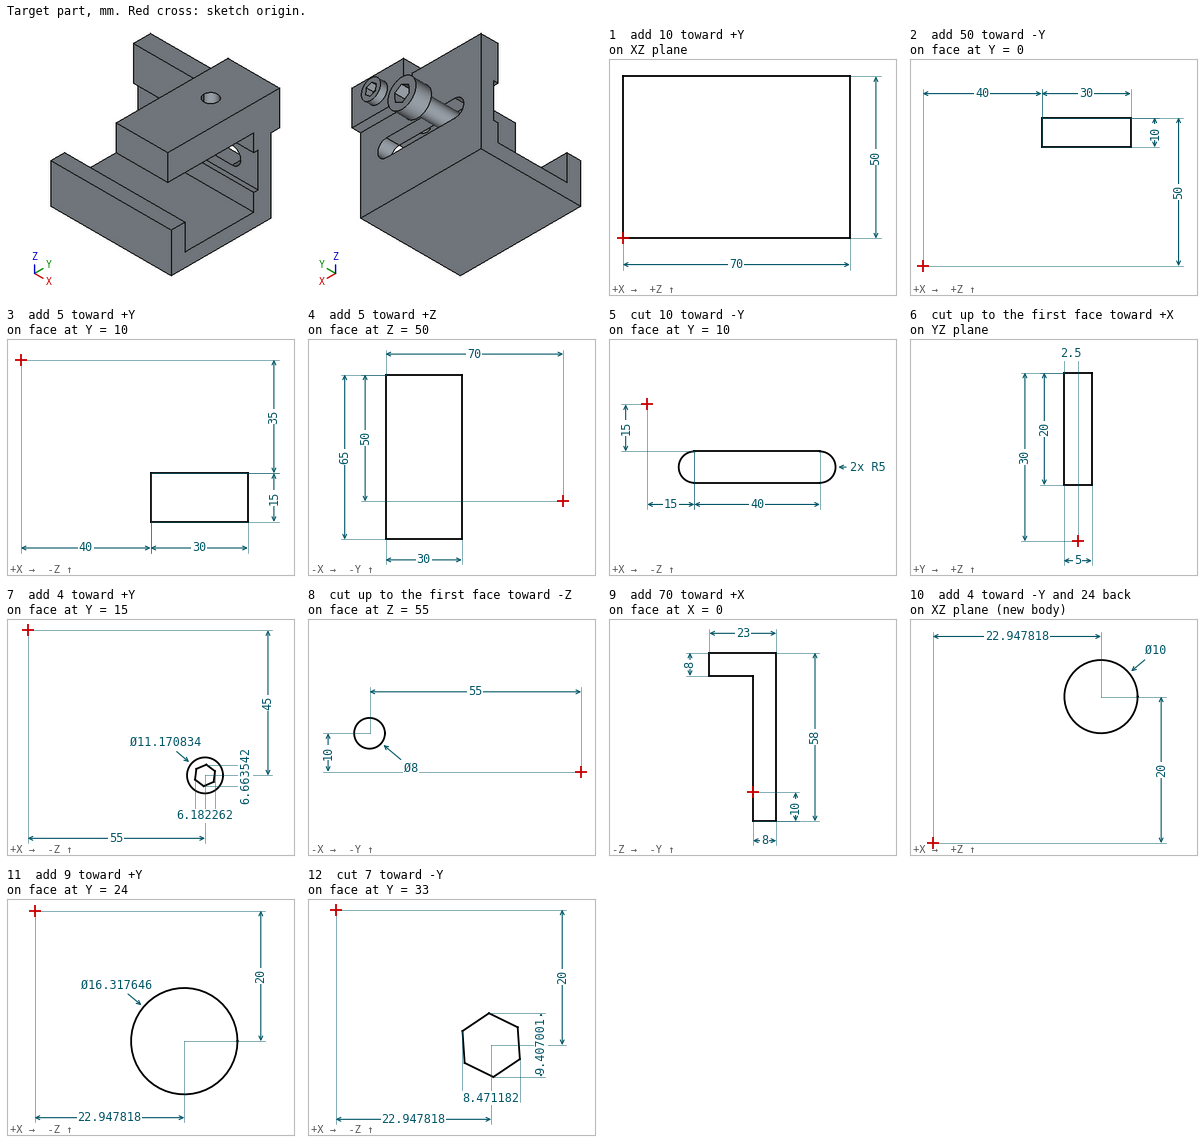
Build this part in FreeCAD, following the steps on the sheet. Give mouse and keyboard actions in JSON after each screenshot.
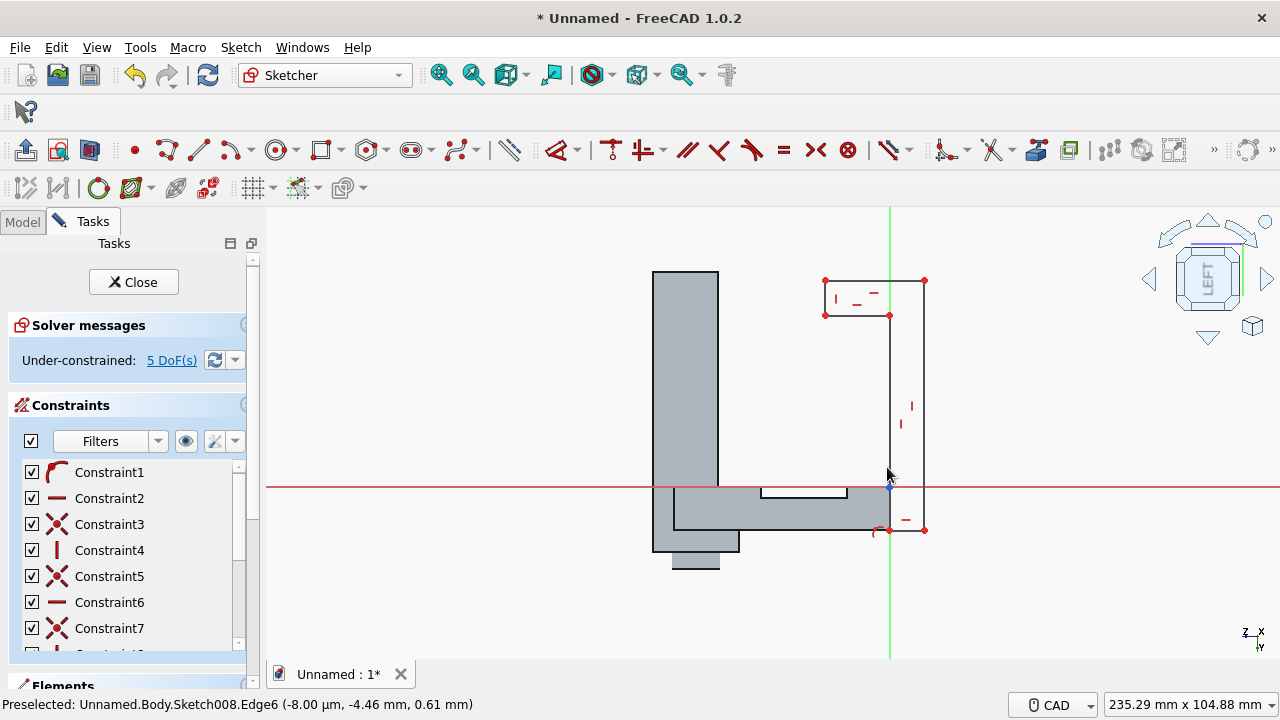
{"action": "left_click", "coordinate": [556, 150]}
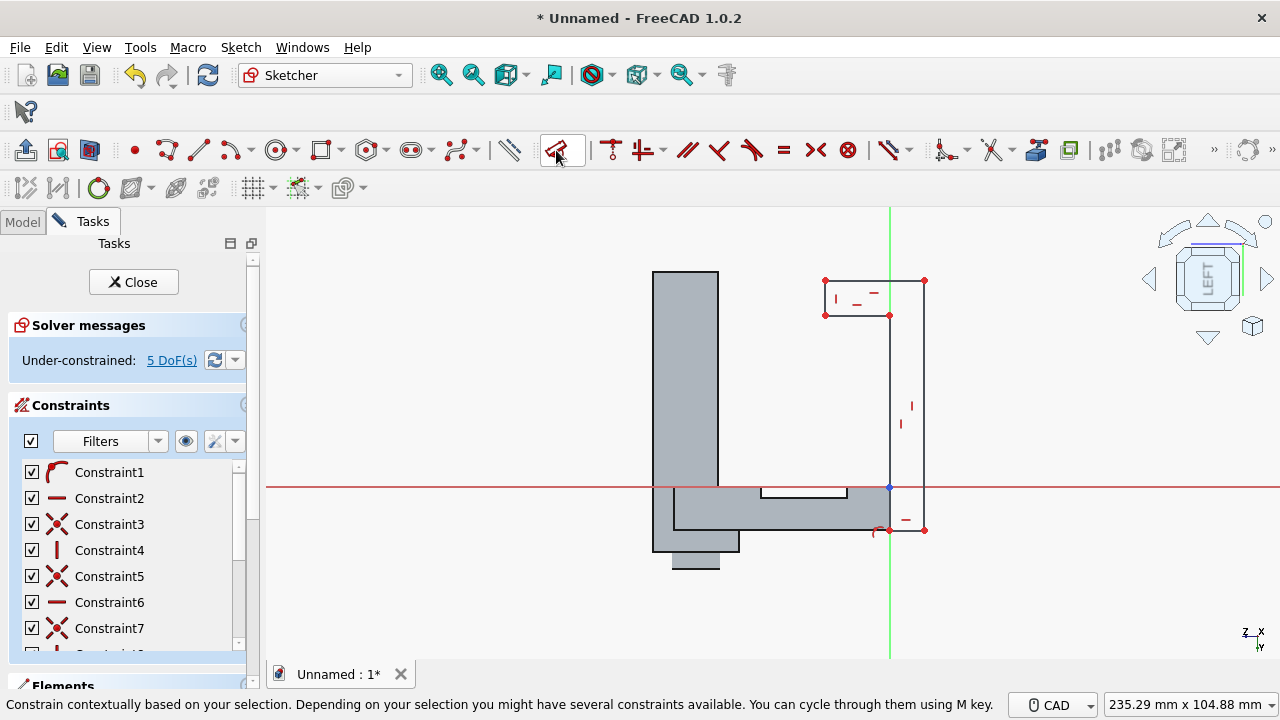
{"action": "scroll", "coordinate": [900, 531], "scroll_direction": "up", "scroll_amount": 2}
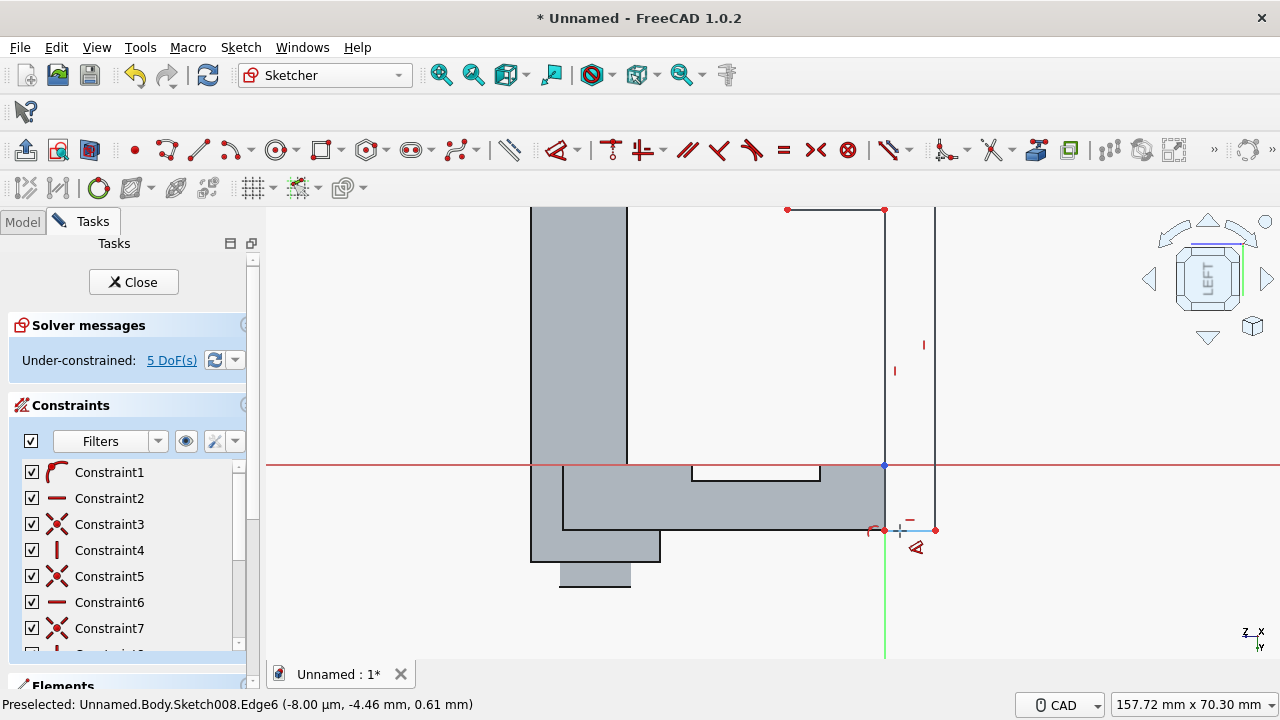
{"action": "left_click", "coordinate": [900, 531]}
{"action": "left_click", "coordinate": [910, 565]}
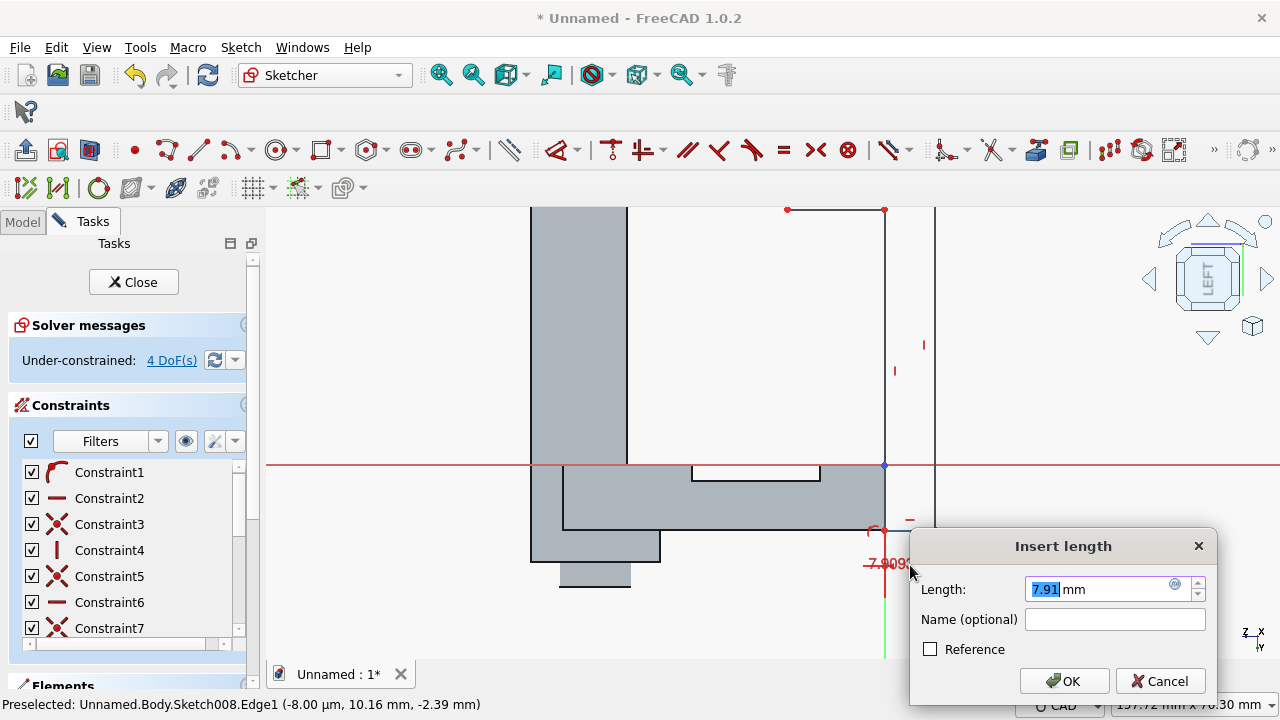
{"action": "type", "text": "8"}
{"action": "key", "text": "Return"}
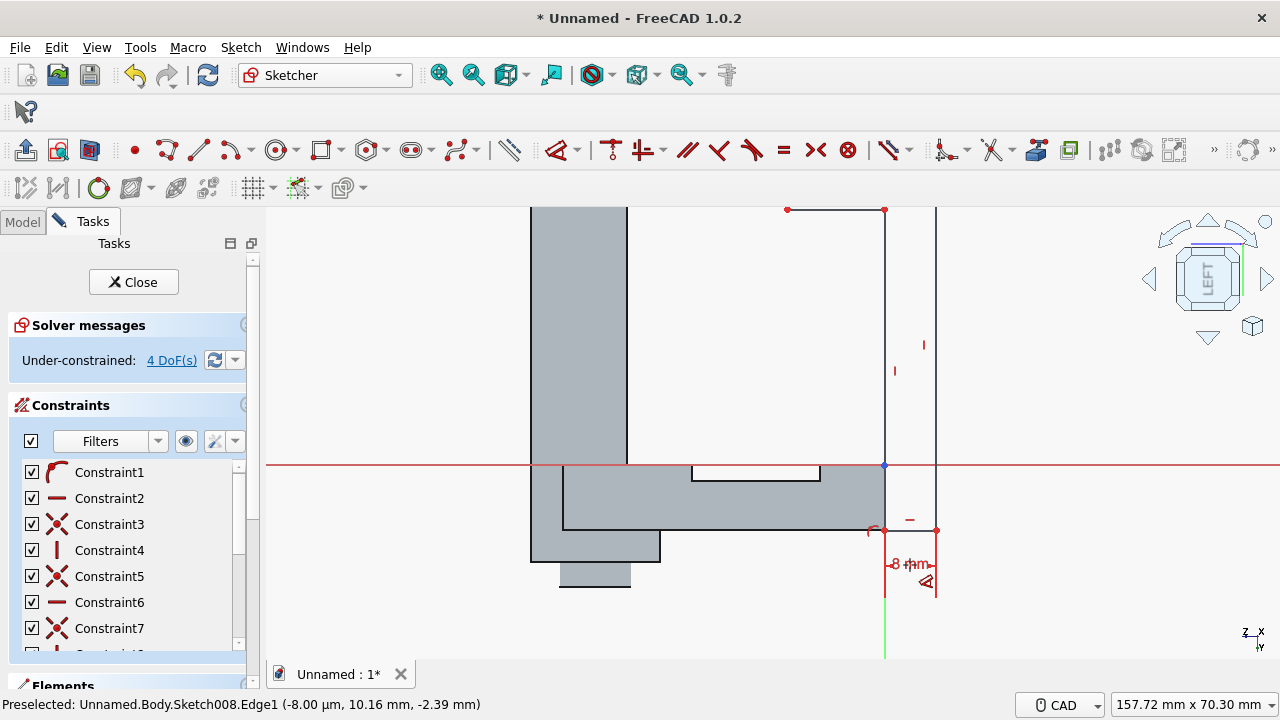
{"action": "scroll", "coordinate": [384, 616], "scroll_direction": "down", "scroll_amount": 2}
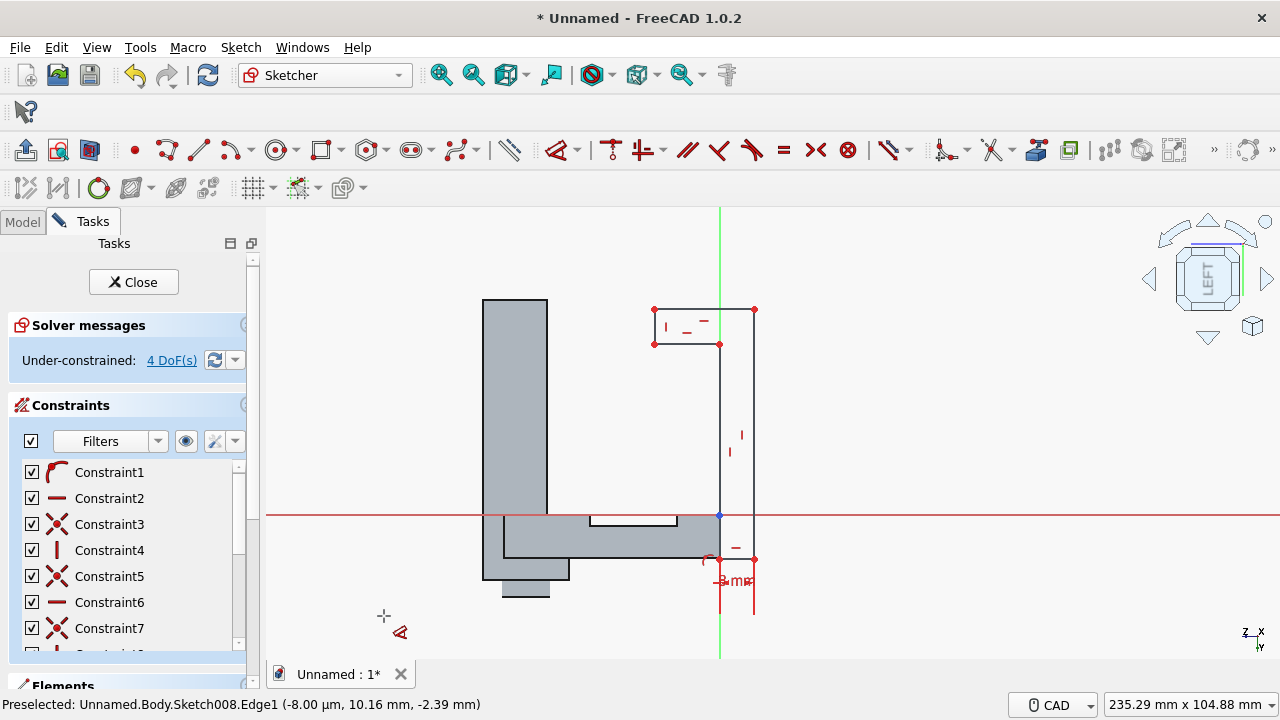
{"action": "scroll", "coordinate": [655, 320], "scroll_direction": "up", "scroll_amount": 2}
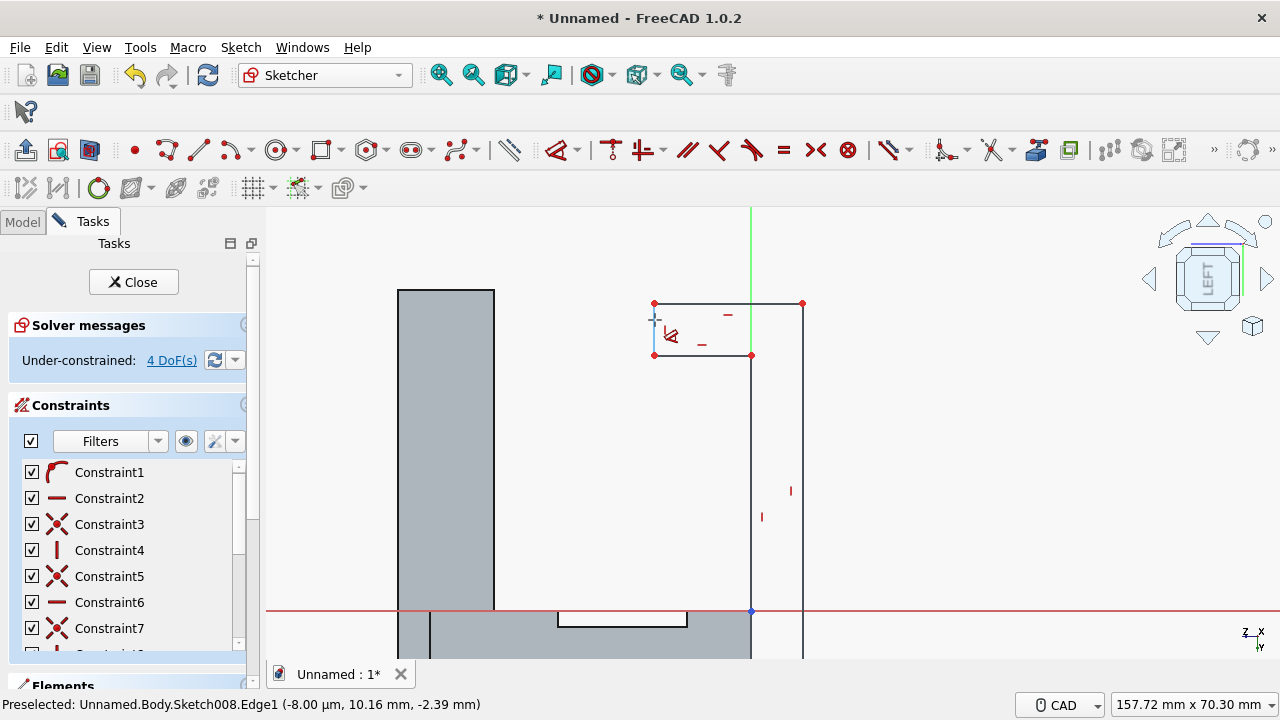
{"action": "left_click", "coordinate": [654, 319]}
{"action": "left_click", "coordinate": [620, 330]}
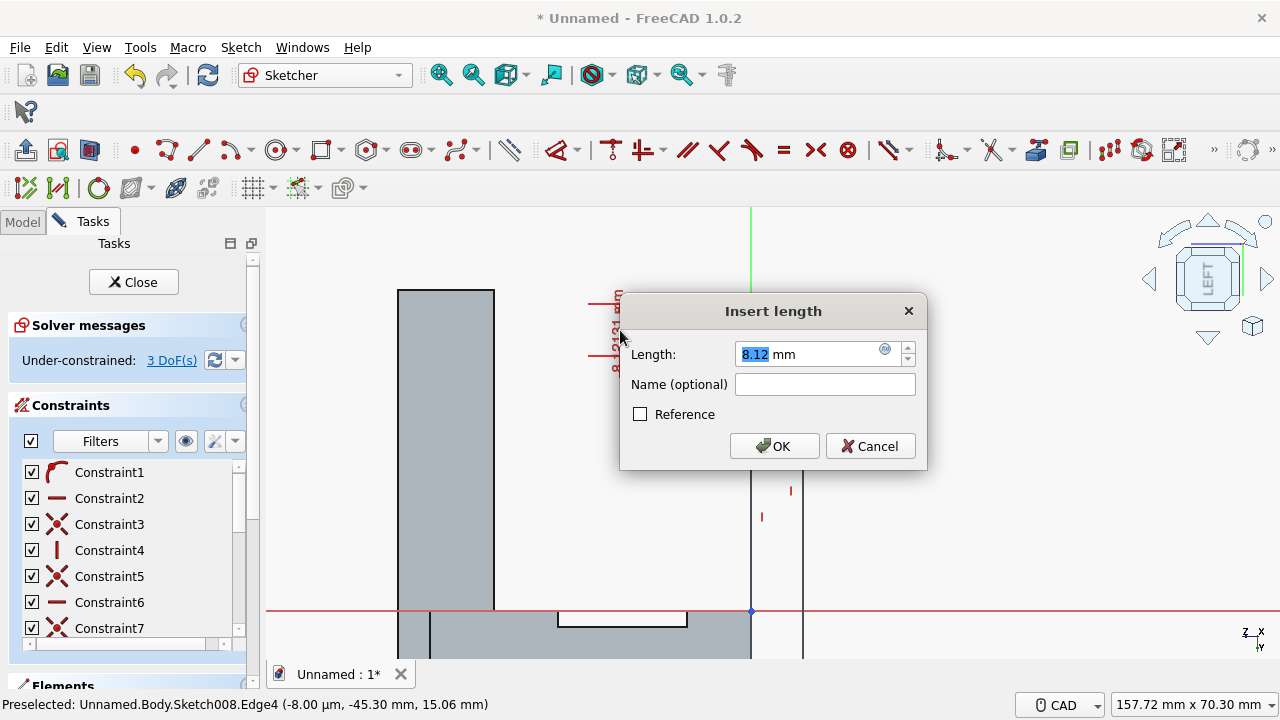
{"action": "type", "text": "8"}
{"action": "key", "text": "Return"}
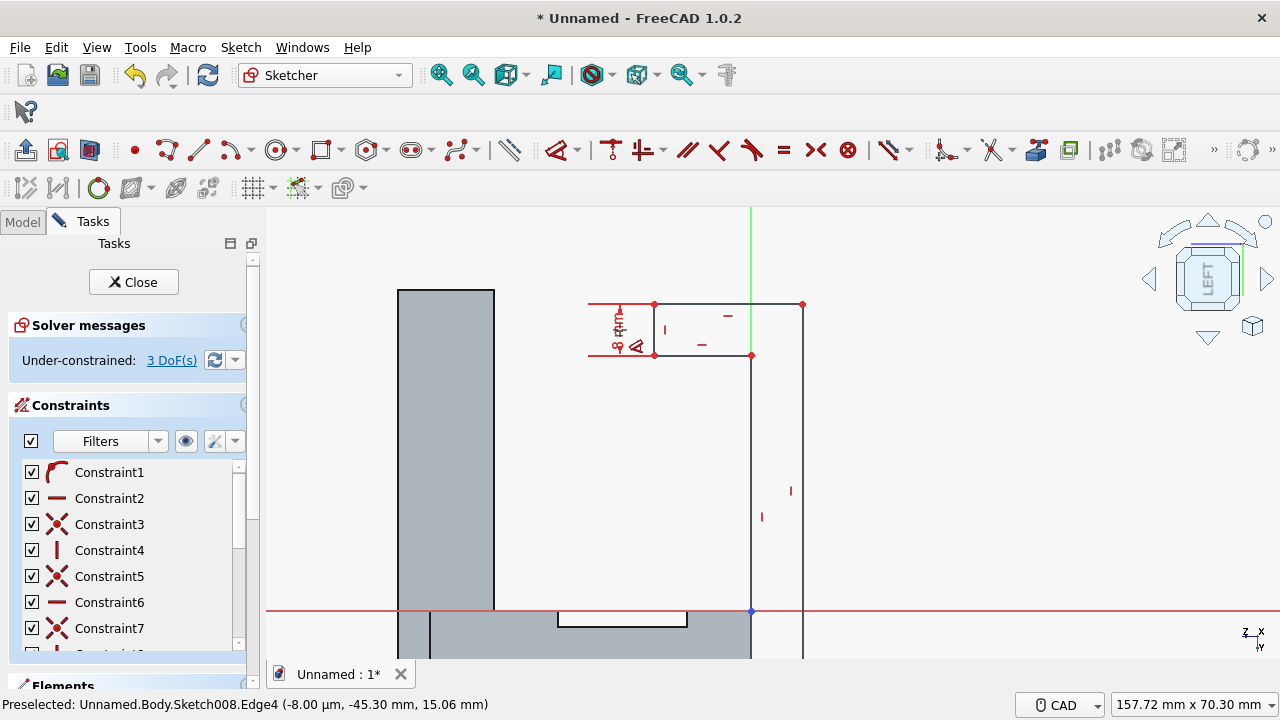
{"action": "left_click", "coordinate": [803, 565]}
{"action": "left_click", "coordinate": [837, 468]}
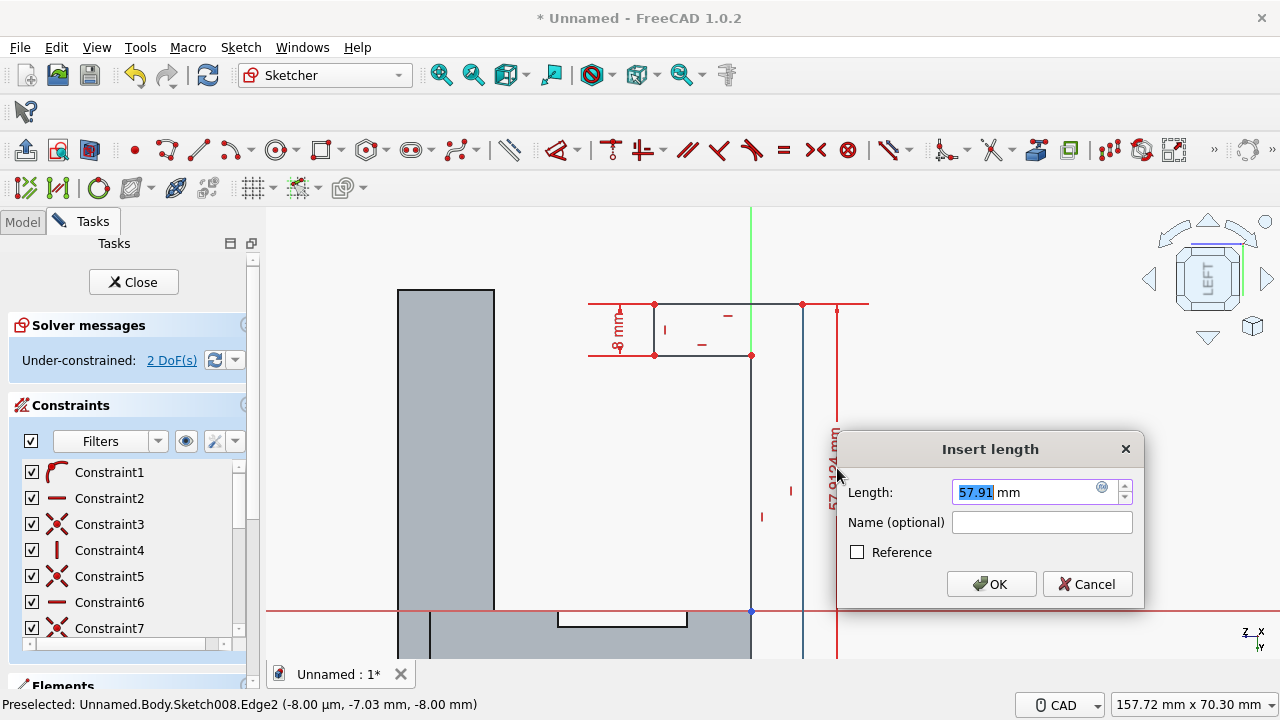
{"action": "type", "text": "58"}
{"action": "key", "text": "Return"}